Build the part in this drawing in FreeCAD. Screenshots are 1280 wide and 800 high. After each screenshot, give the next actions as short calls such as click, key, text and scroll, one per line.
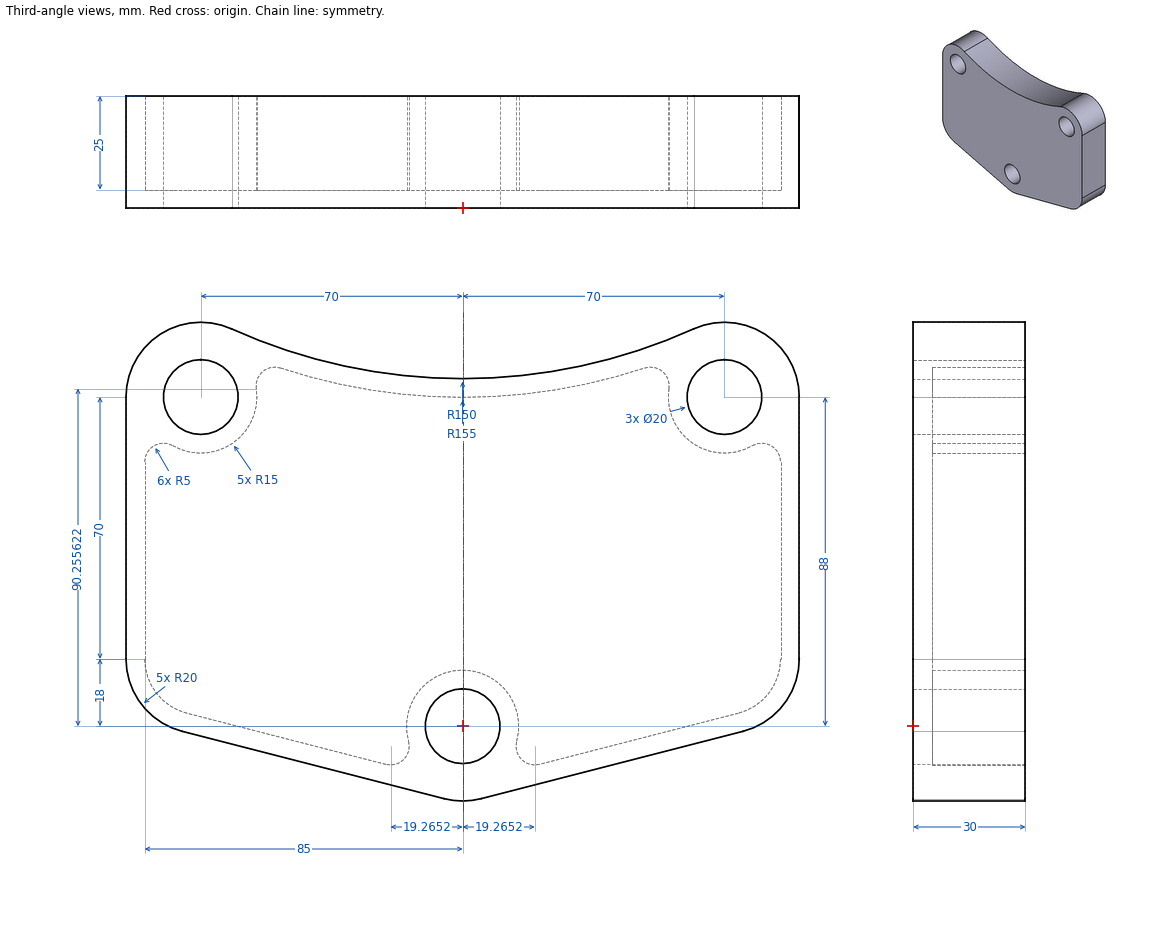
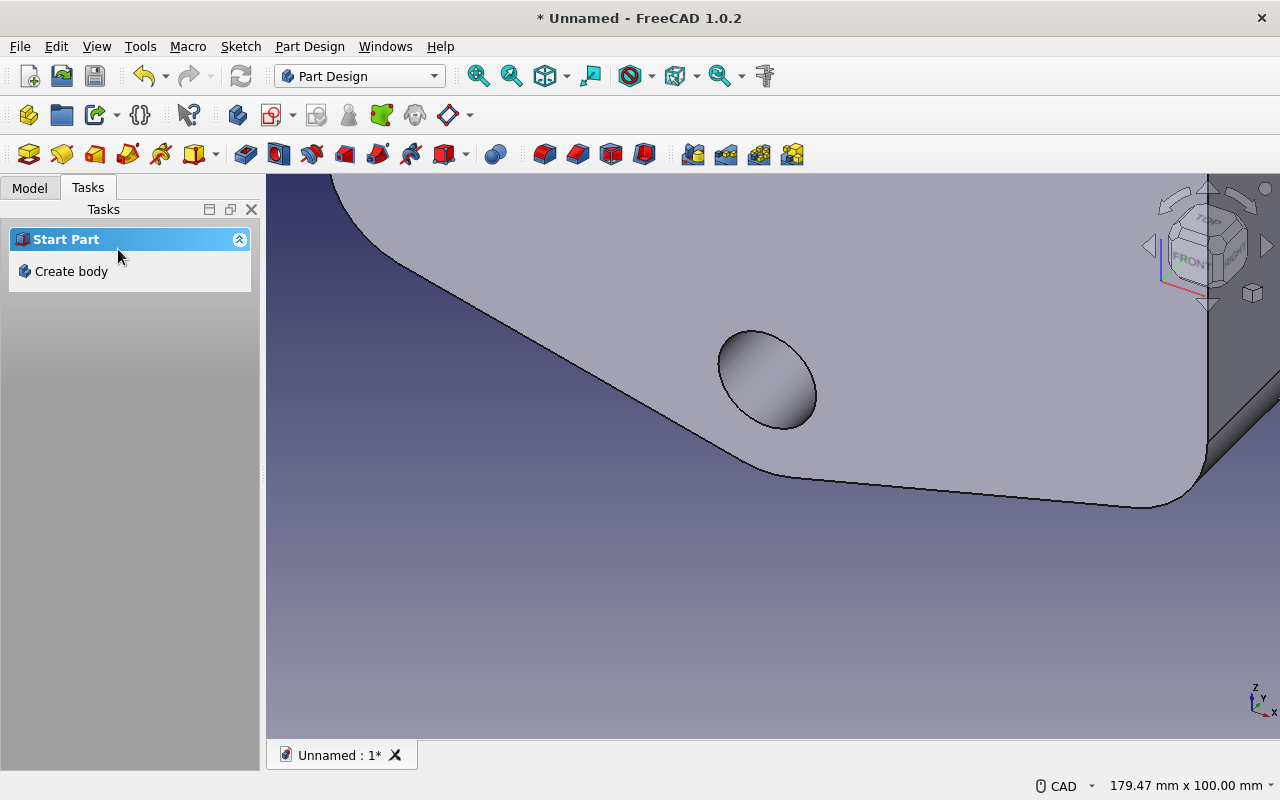
click(479, 76)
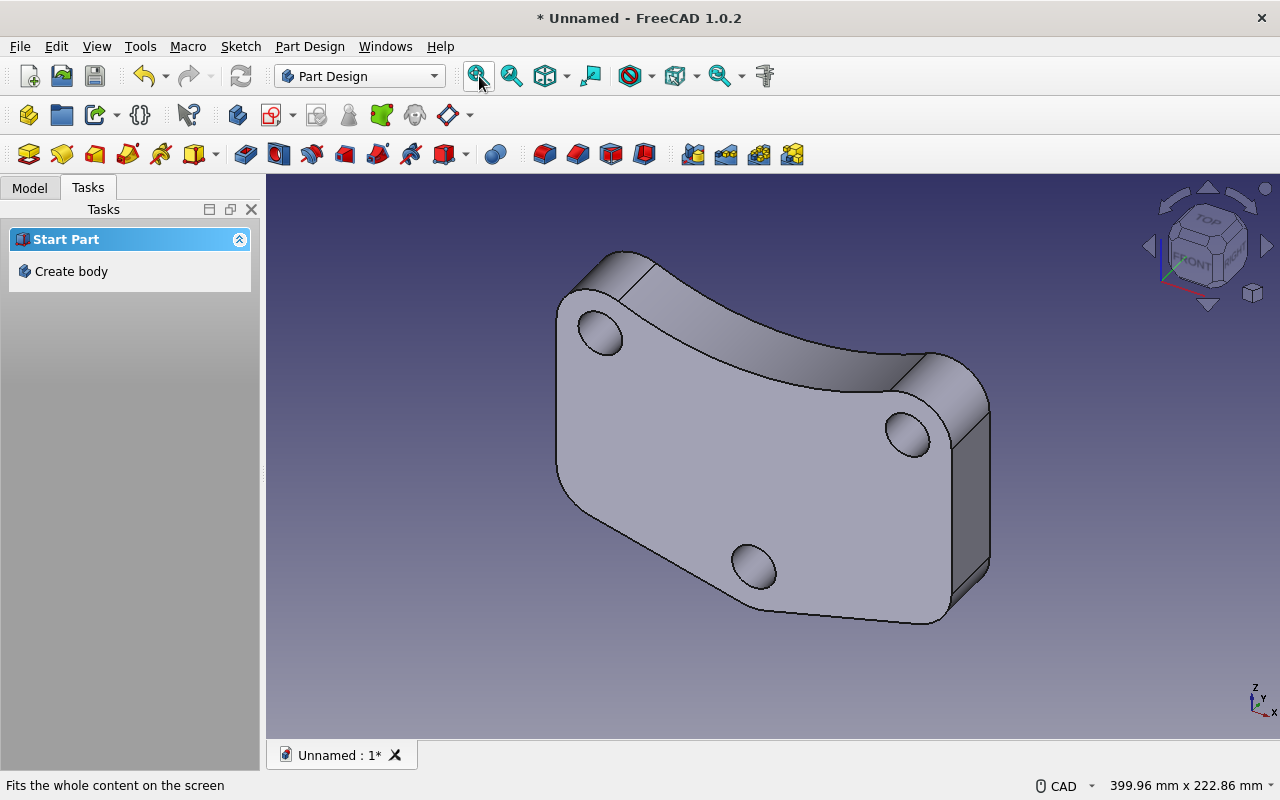
key(4)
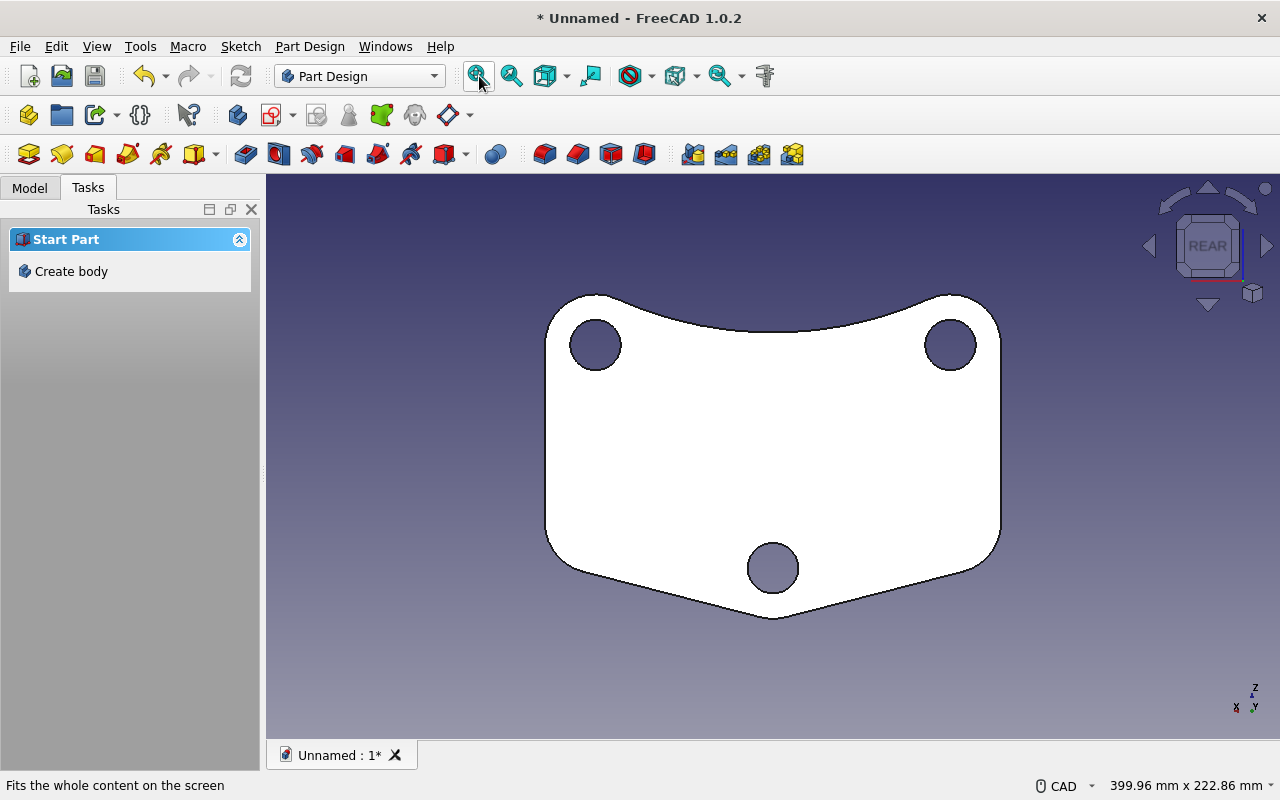
click(708, 456)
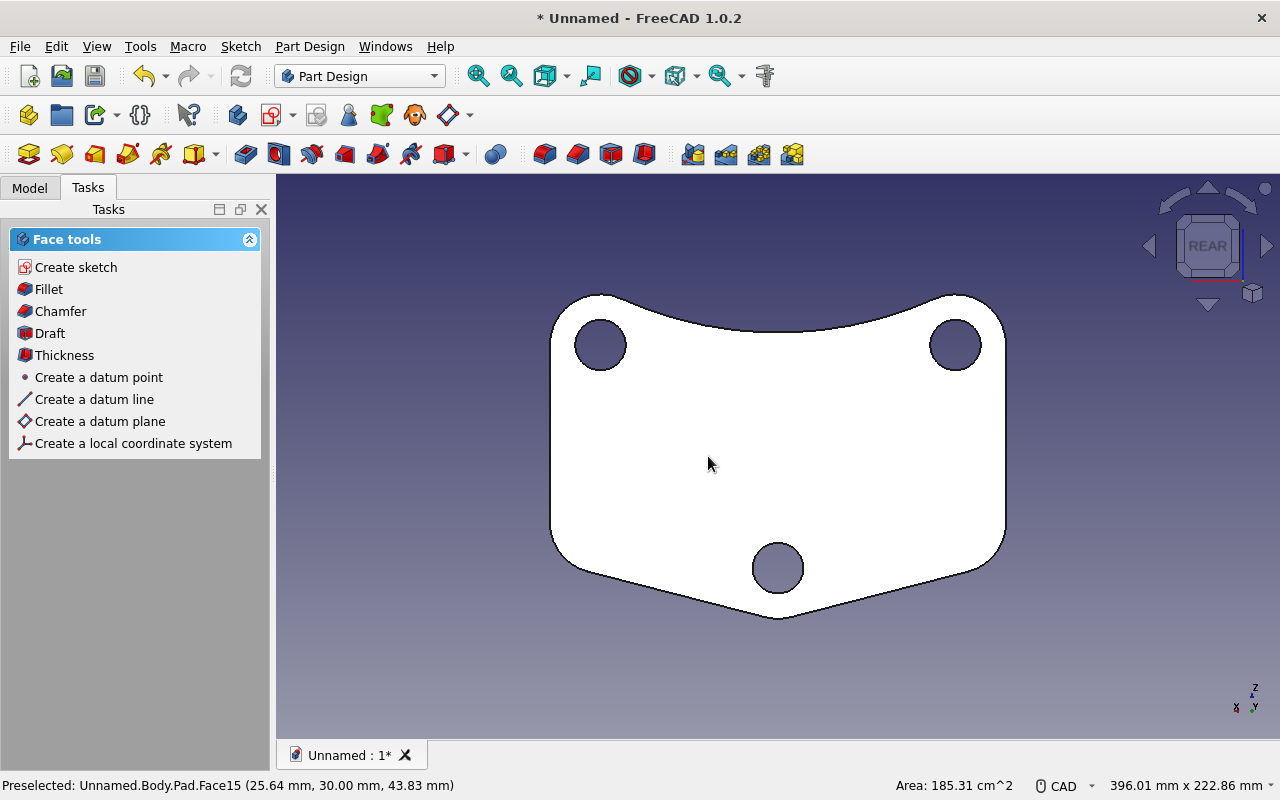
click(270, 116)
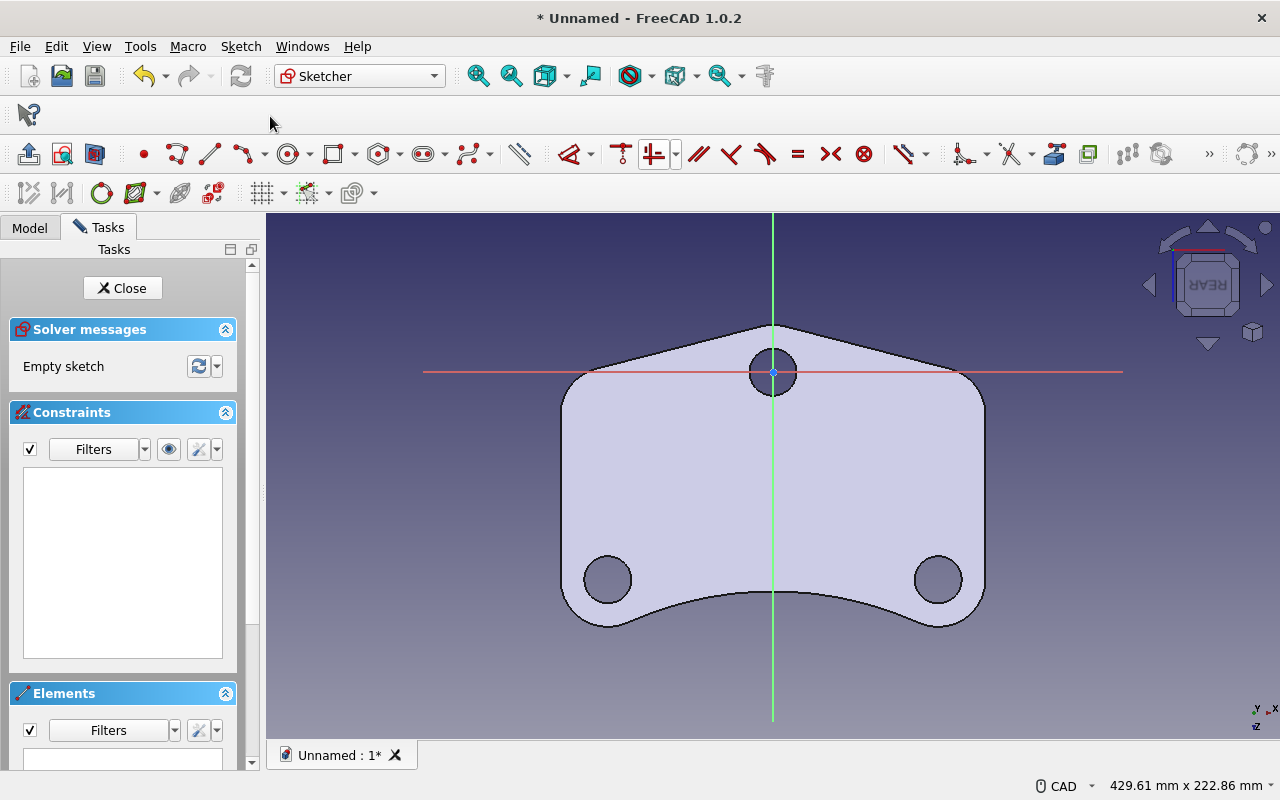
click(210, 154)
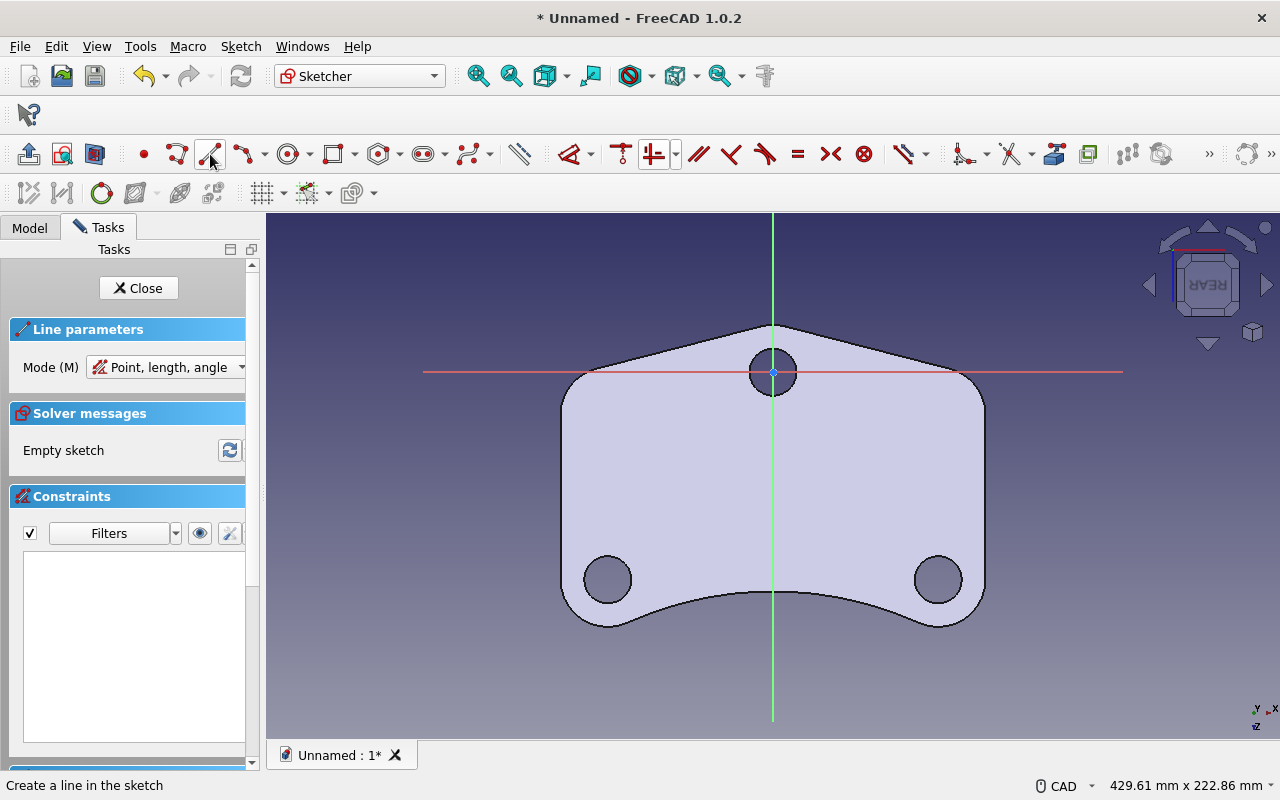
click(572, 415)
click(572, 539)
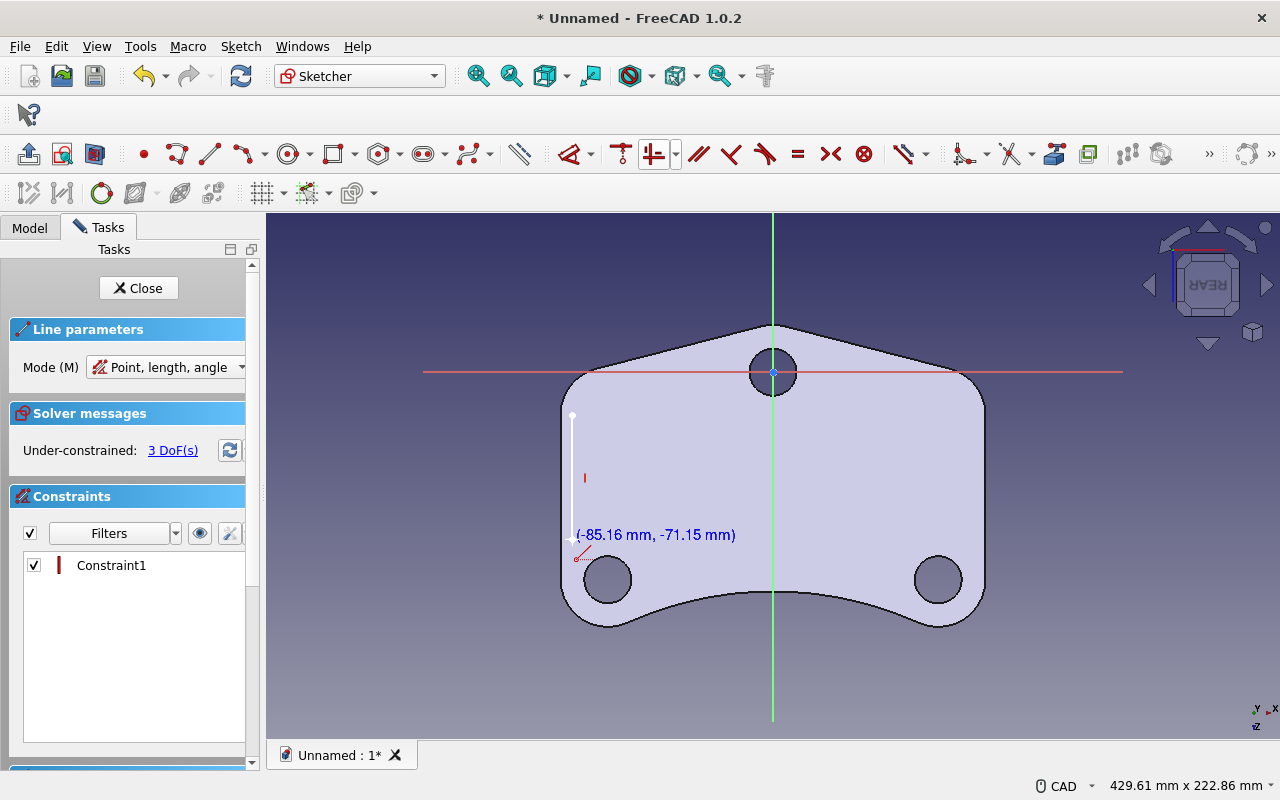
click(974, 539)
click(974, 415)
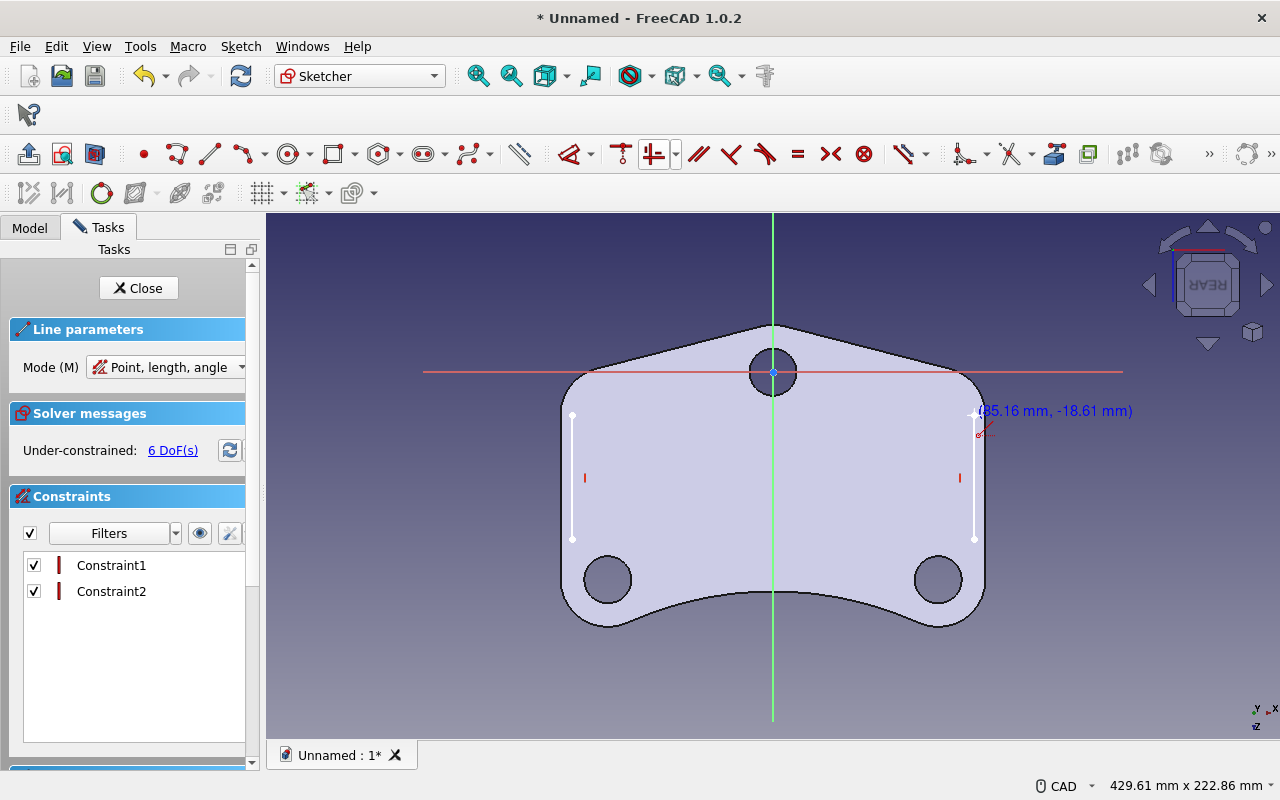
scroll(947, 380, up, 4)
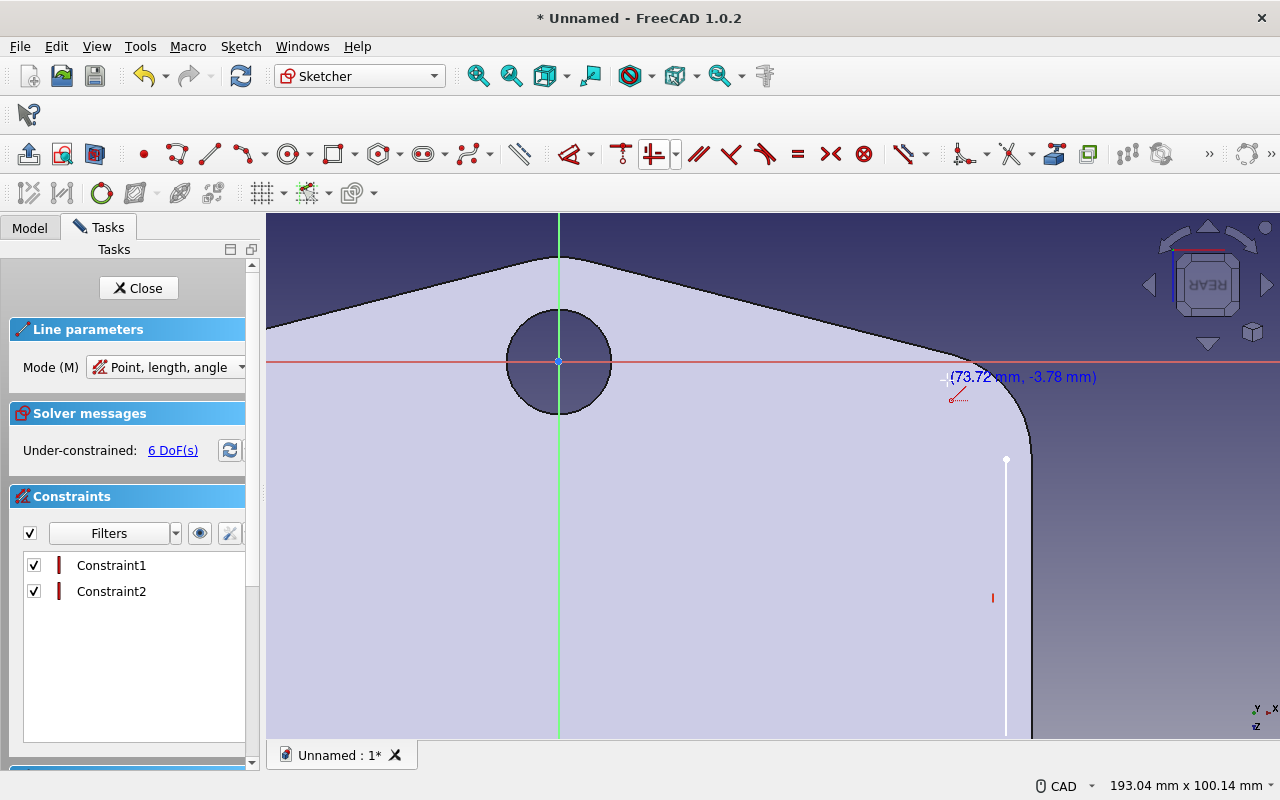
click(946, 380)
click(667, 308)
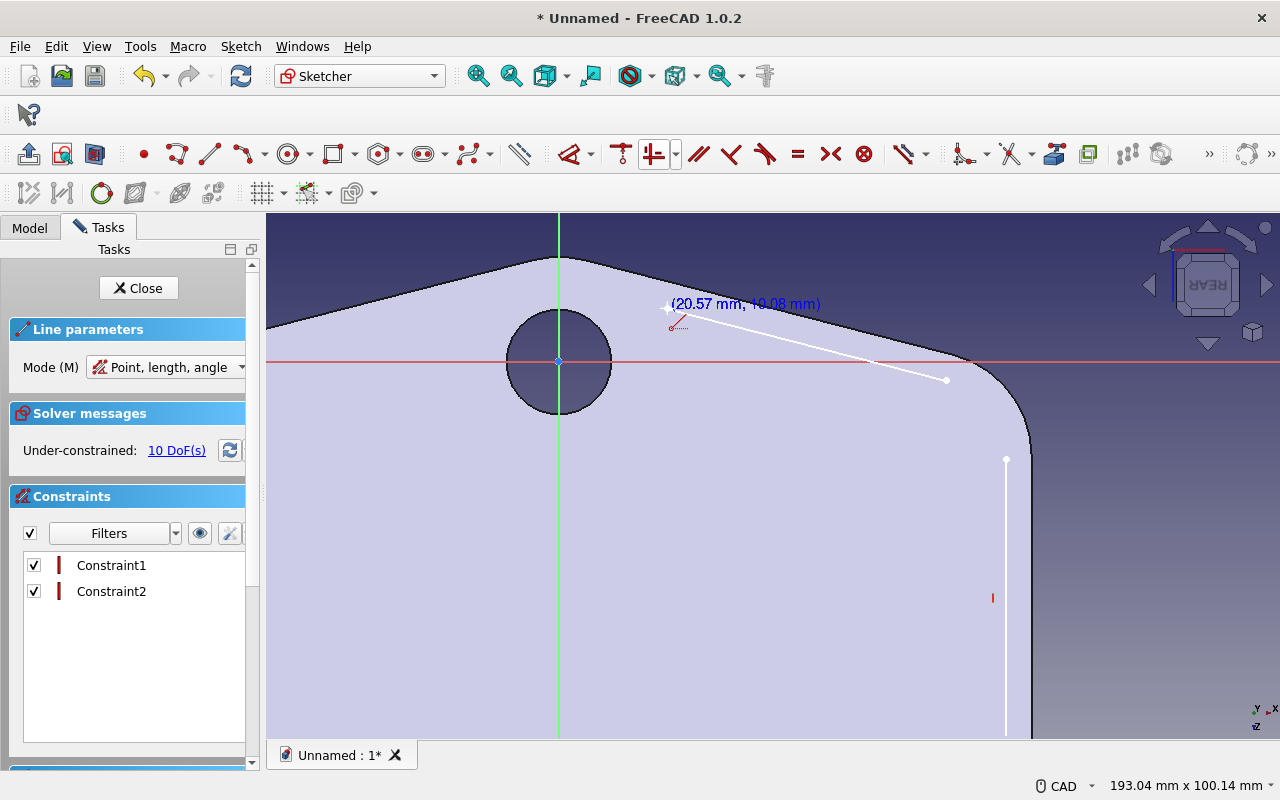
click(451, 308)